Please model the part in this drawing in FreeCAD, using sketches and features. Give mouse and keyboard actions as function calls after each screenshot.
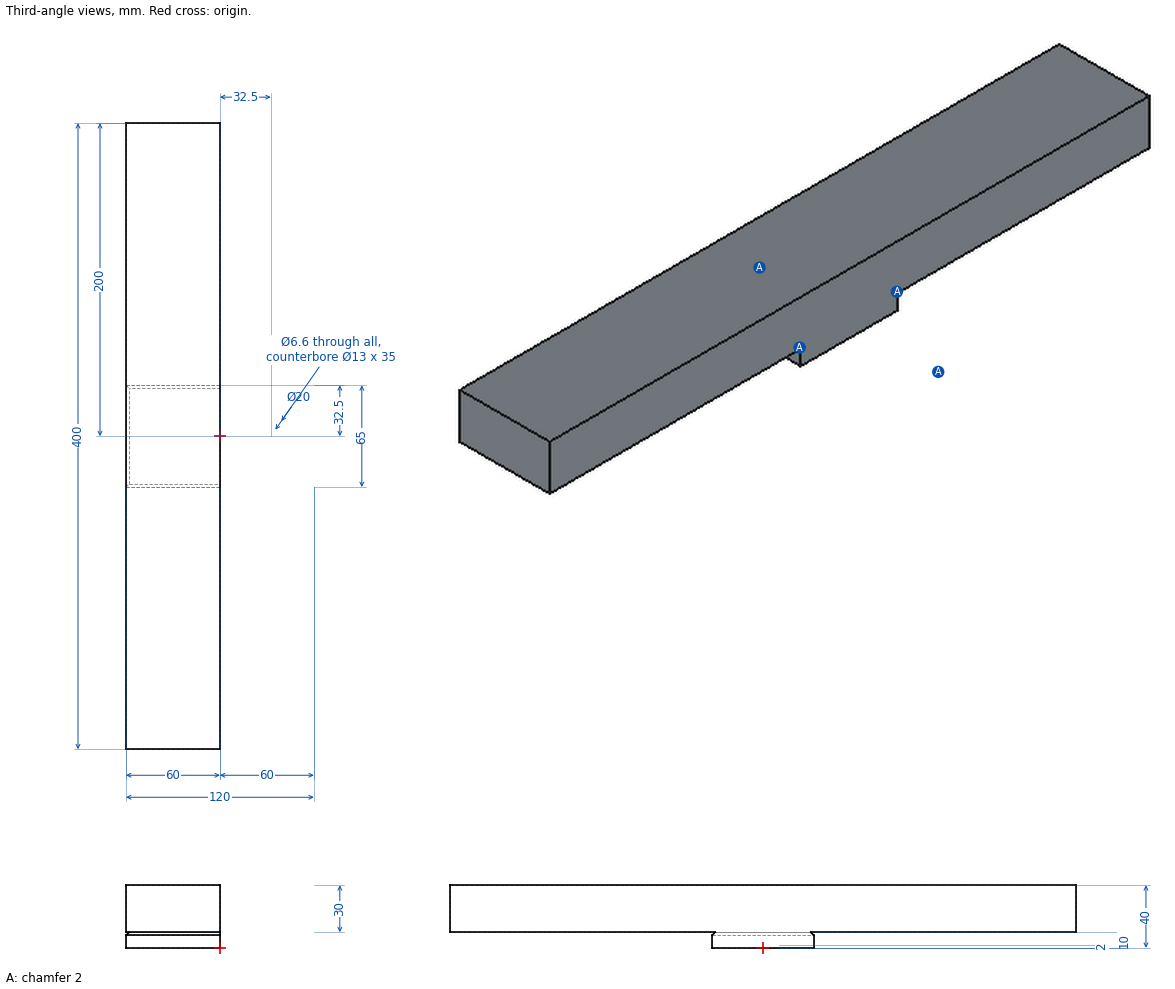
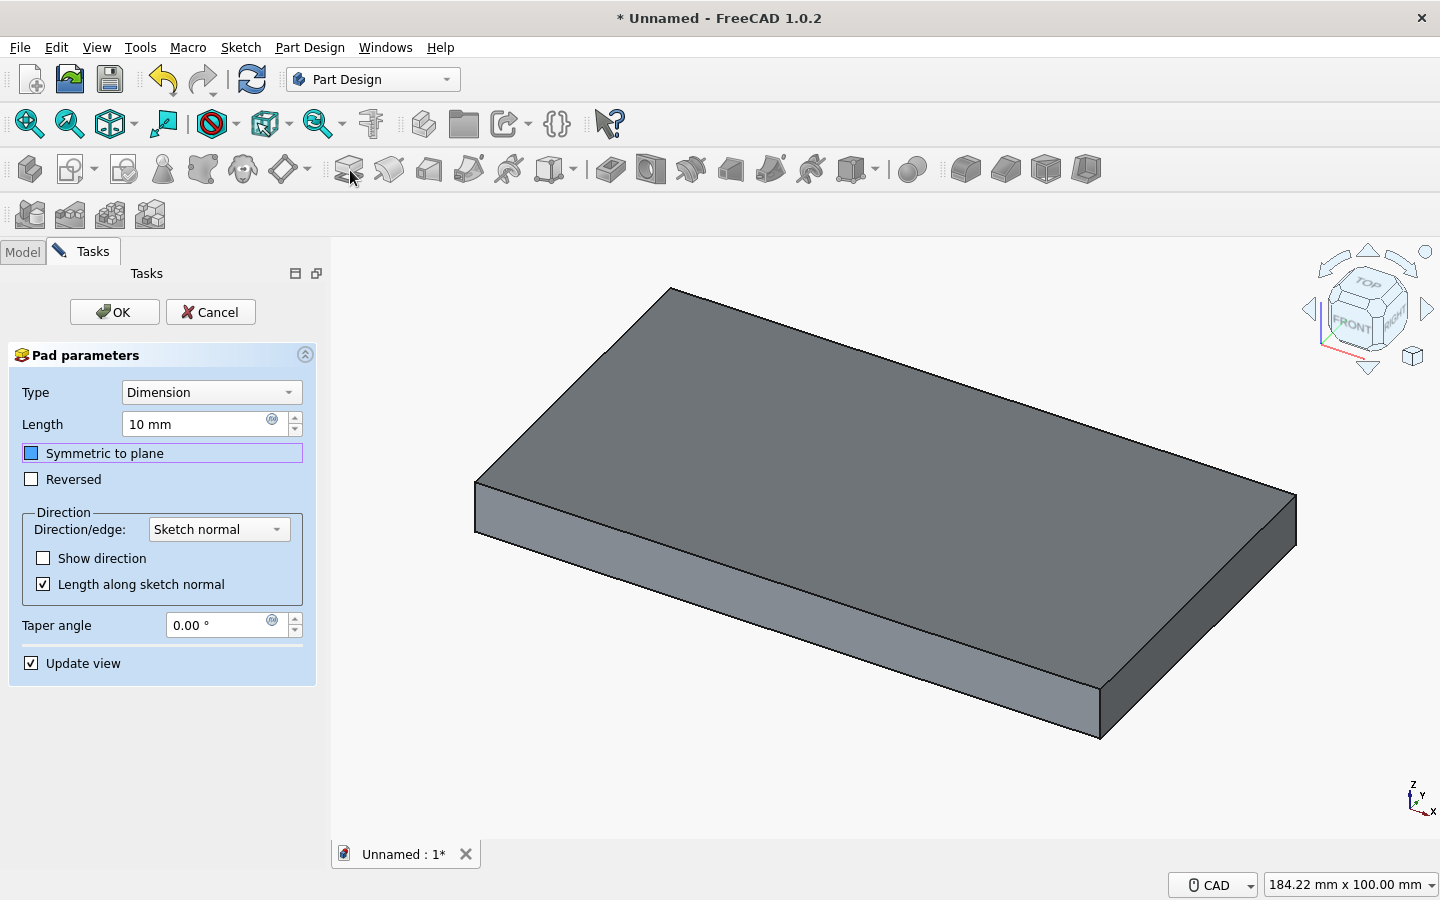
click(115, 312)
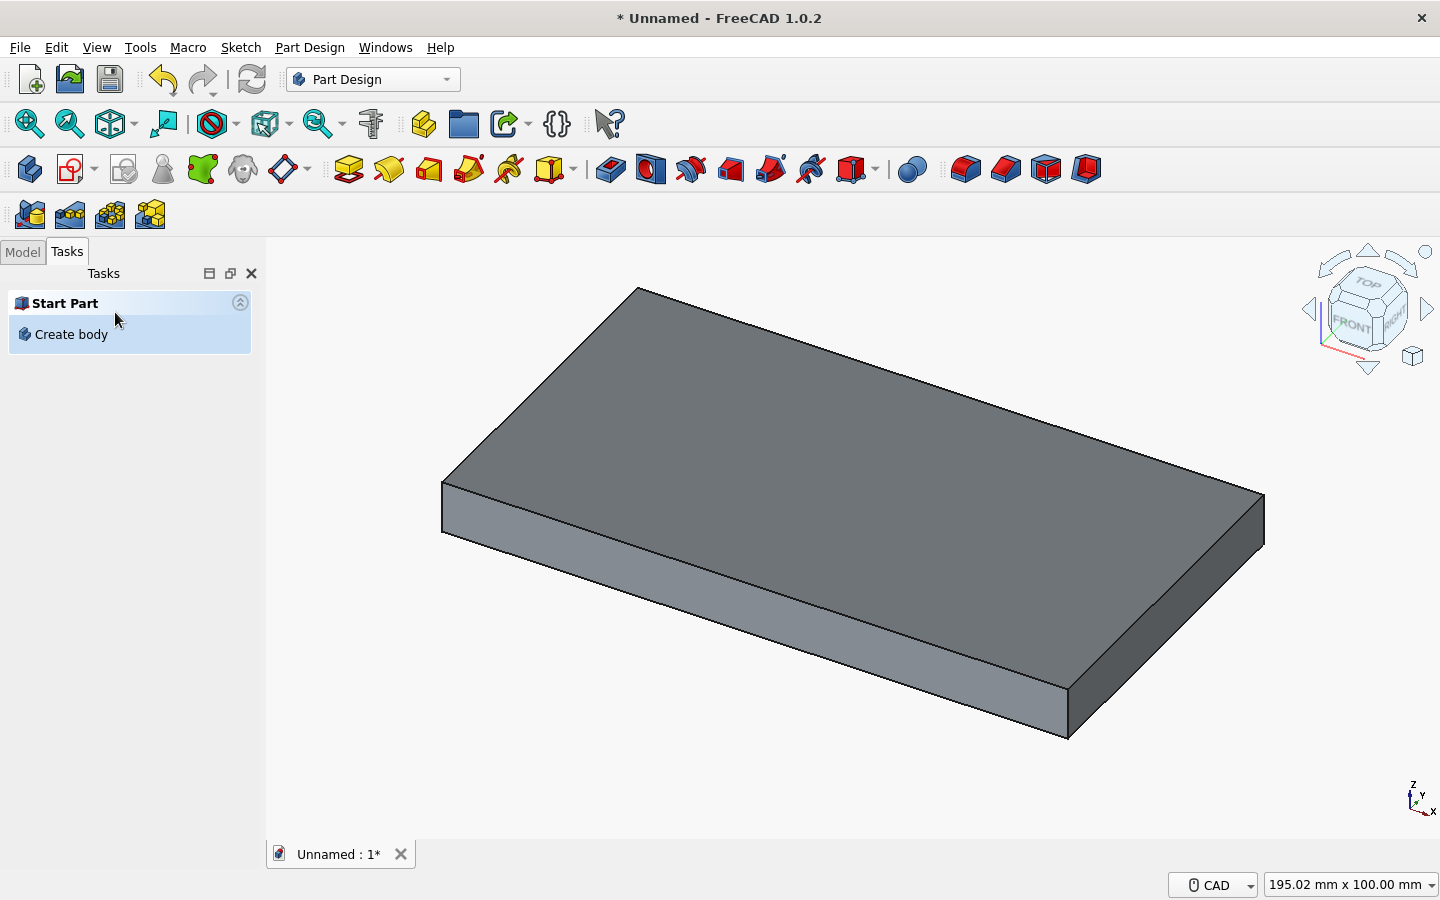
click(942, 517)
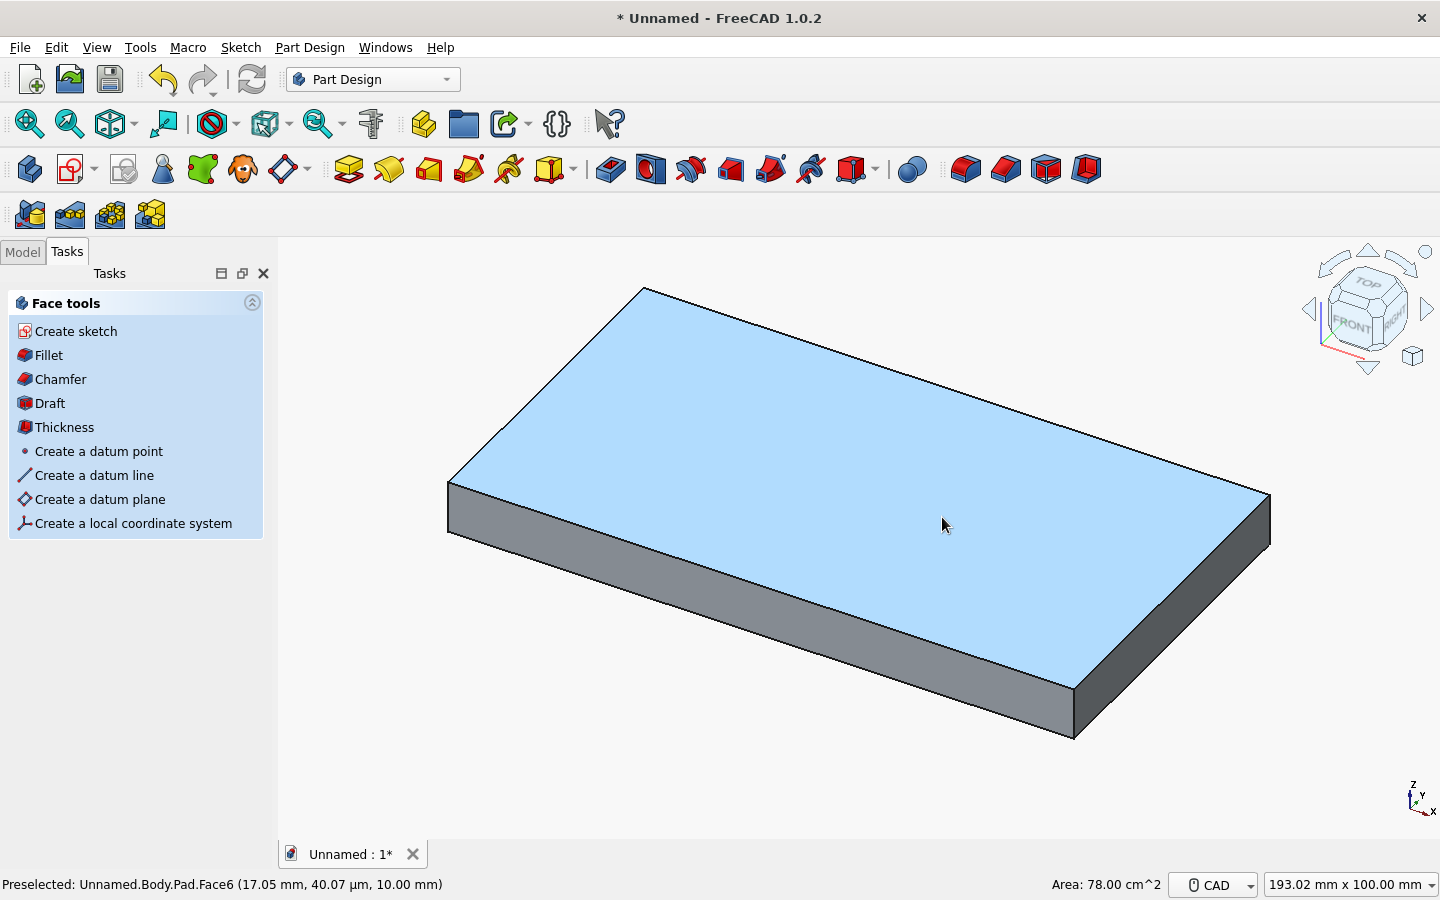
click(1006, 170)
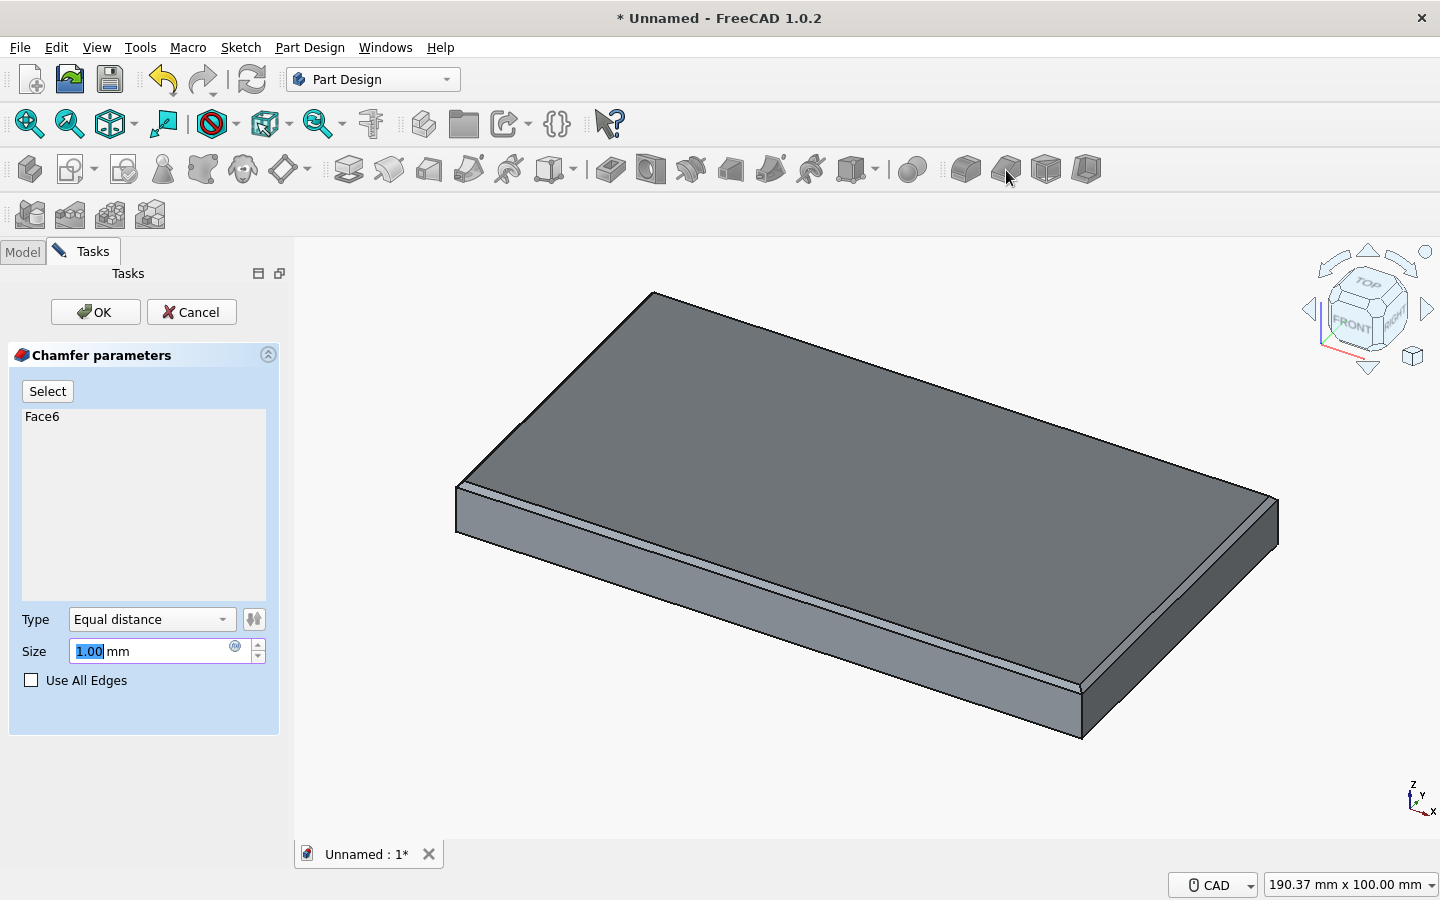
text(2)
key(Tab)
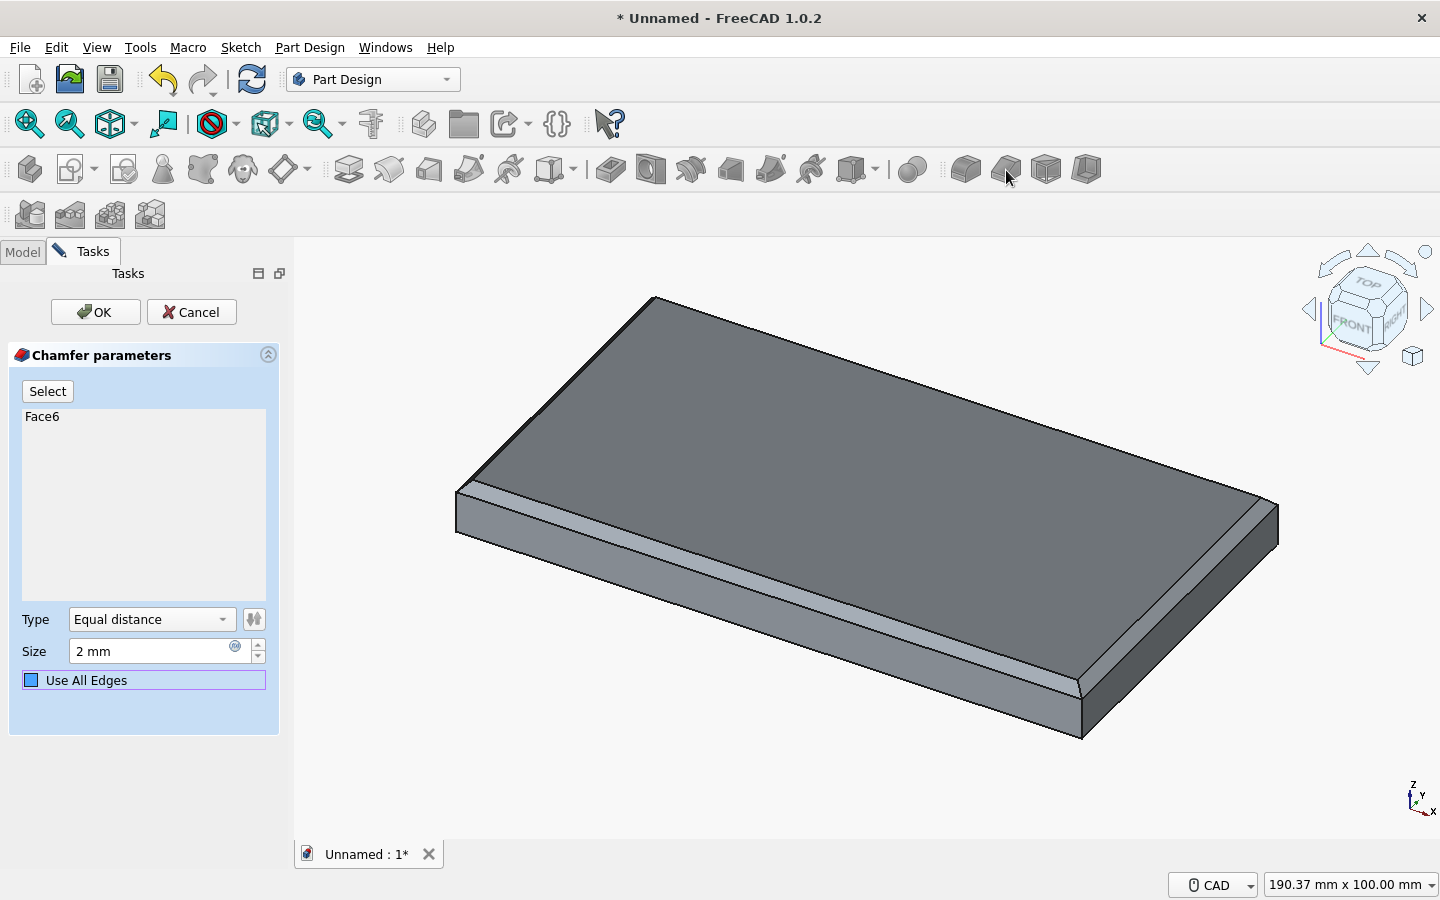
click(96, 312)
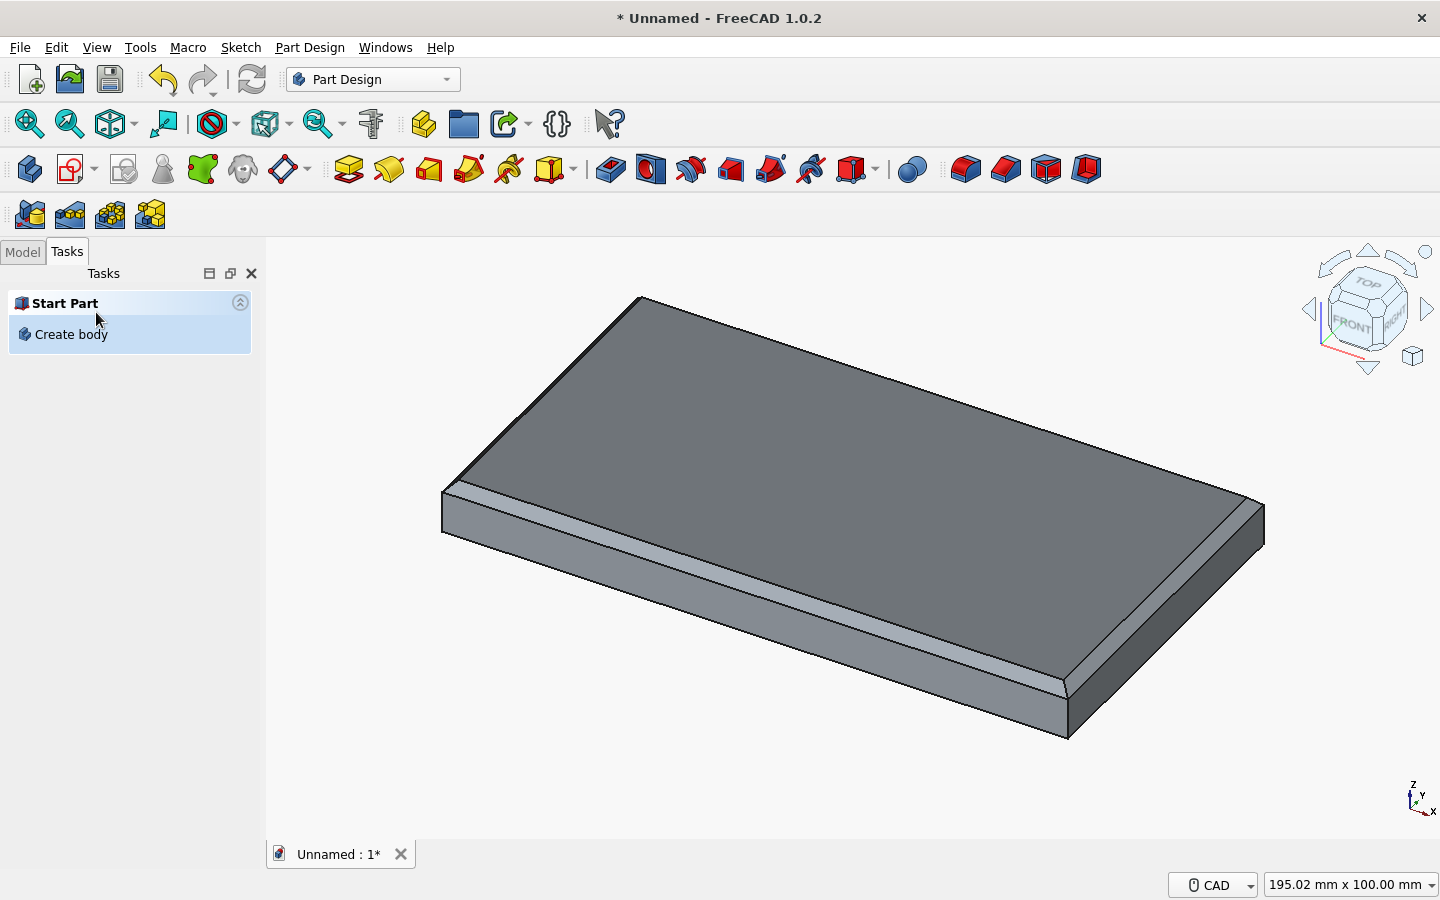
click(939, 516)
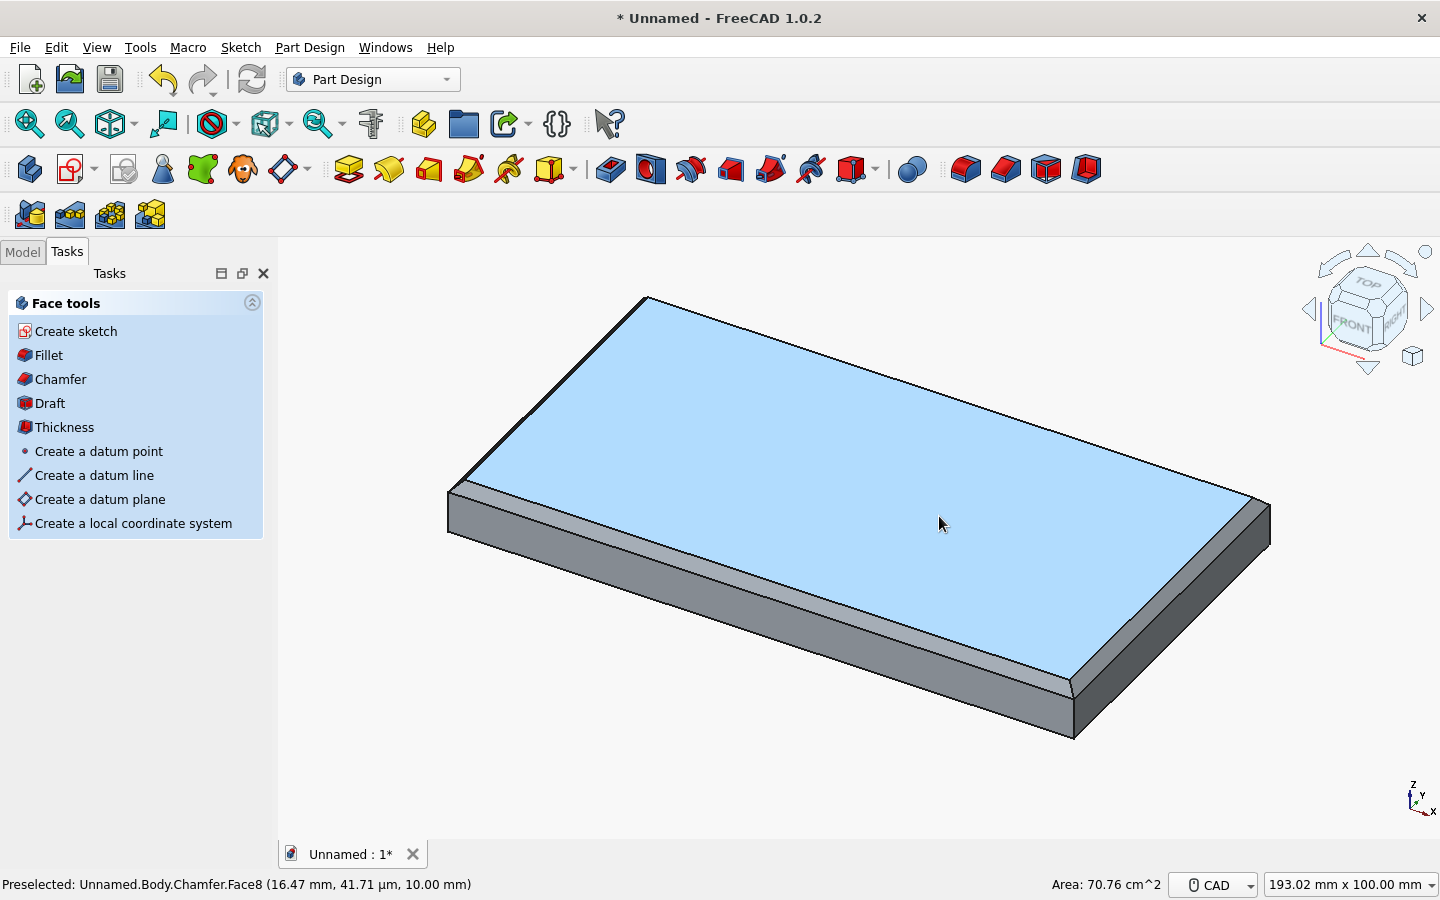
click(70, 170)